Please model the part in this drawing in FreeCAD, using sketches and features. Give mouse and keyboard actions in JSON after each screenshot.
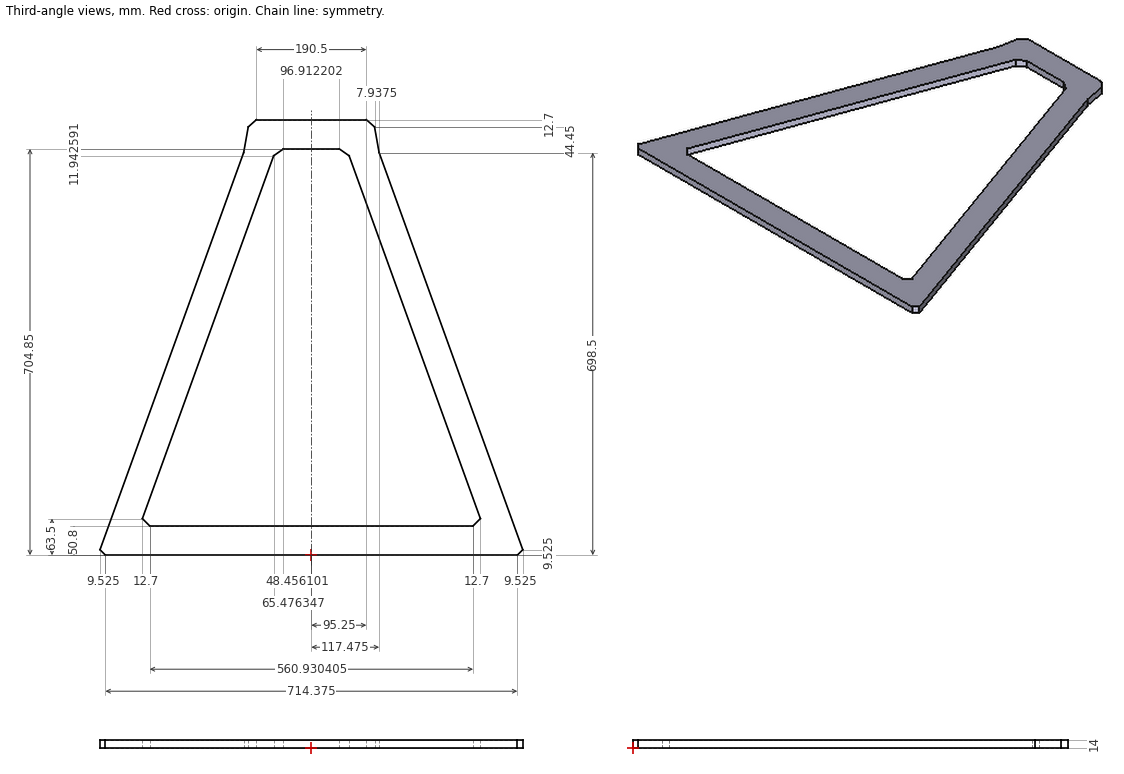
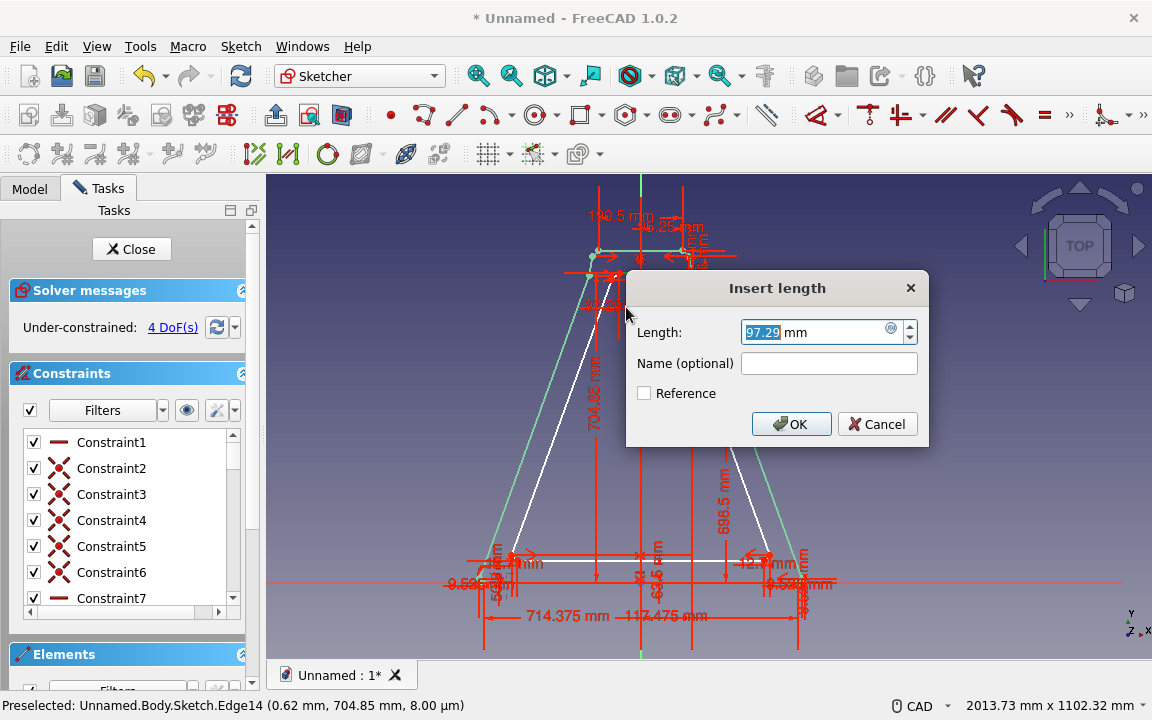
{"action": "type", "text": "96.912202"}
{"action": "key", "text": "Return"}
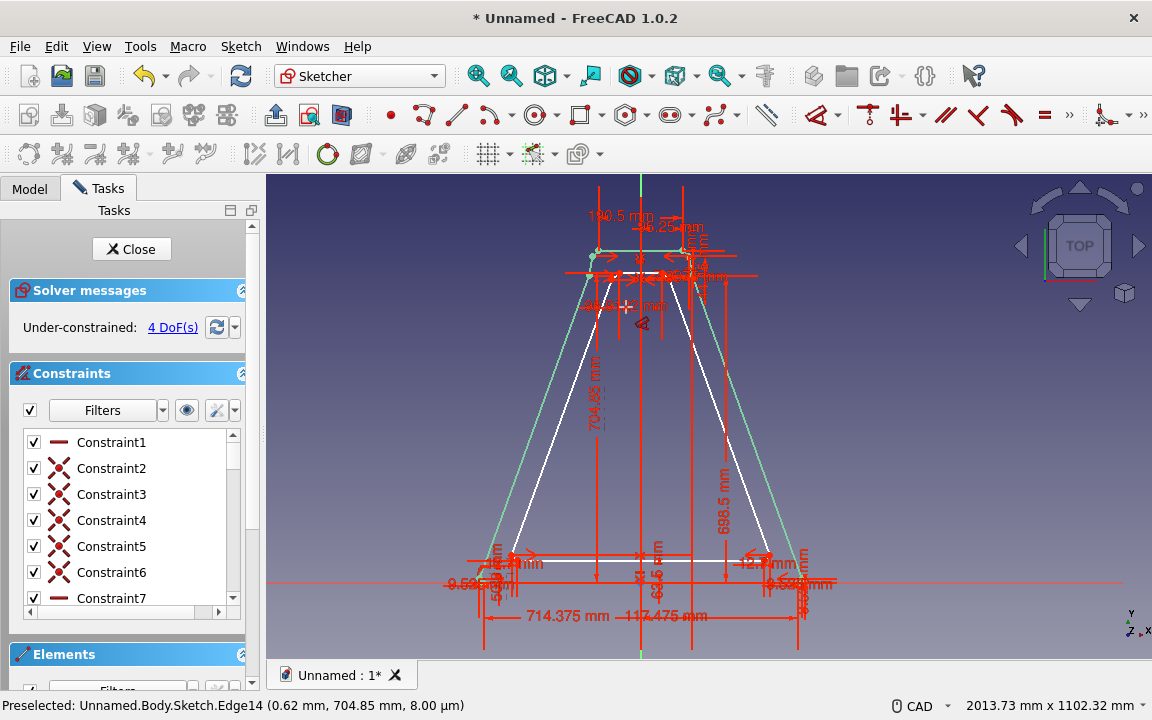
{"action": "left_click", "coordinate": [690, 561]}
{"action": "left_click", "coordinate": [584, 527]}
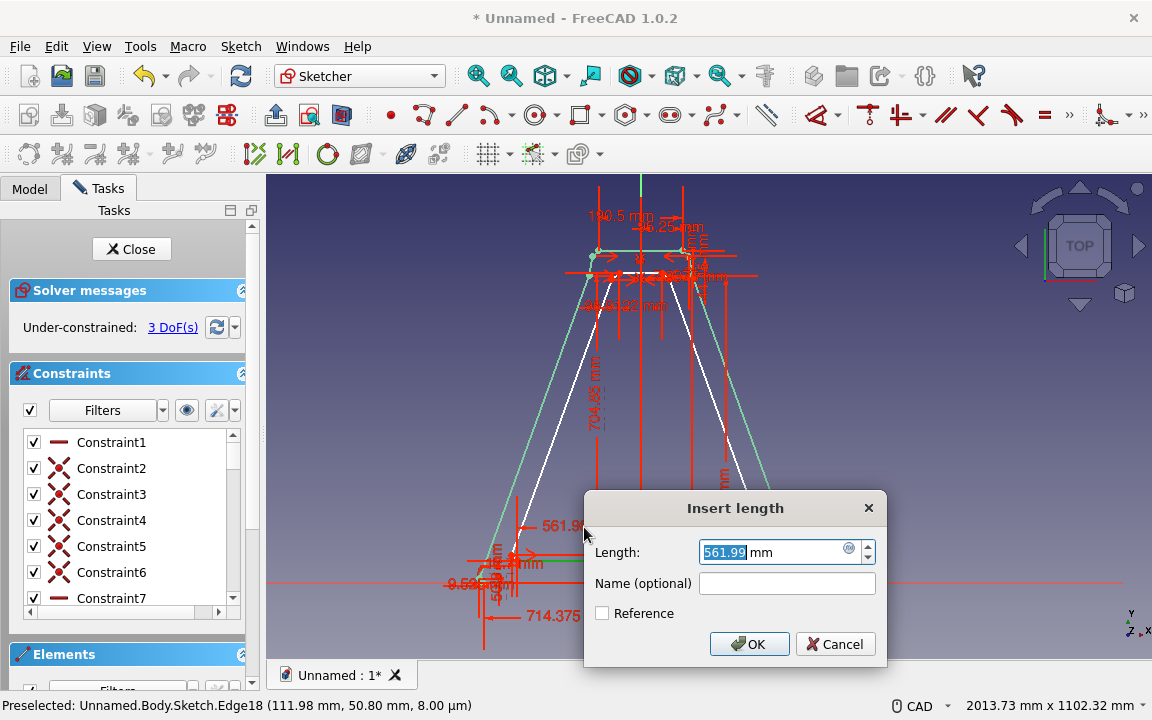
{"action": "type", "text": "560.930405"}
{"action": "key", "text": "Return"}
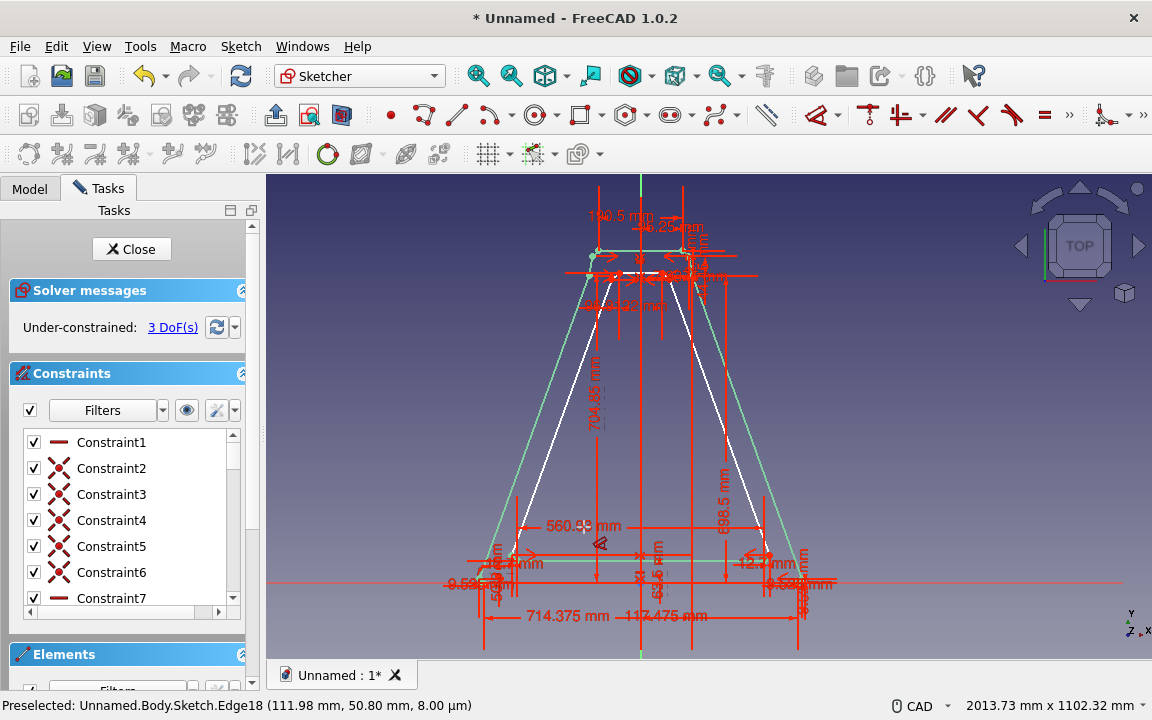
{"action": "scroll", "coordinate": [612, 280], "scroll_direction": "up", "scroll_amount": 2}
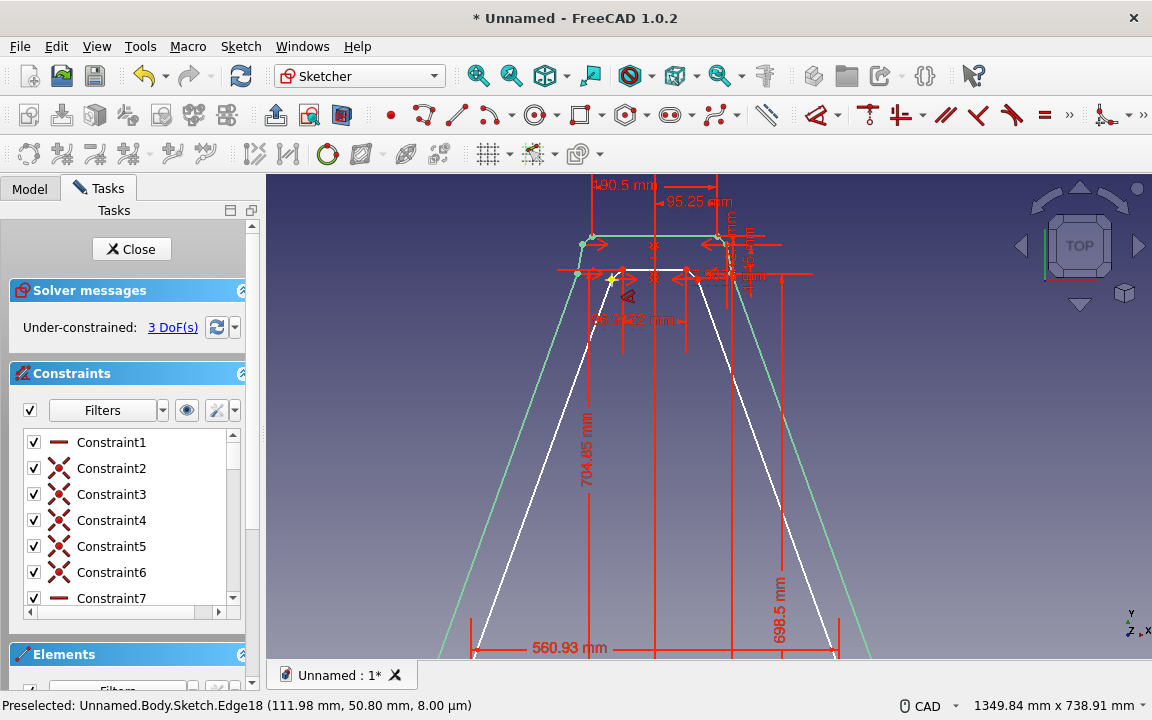
{"action": "left_click", "coordinate": [612, 279]}
{"action": "left_click", "coordinate": [623, 221]}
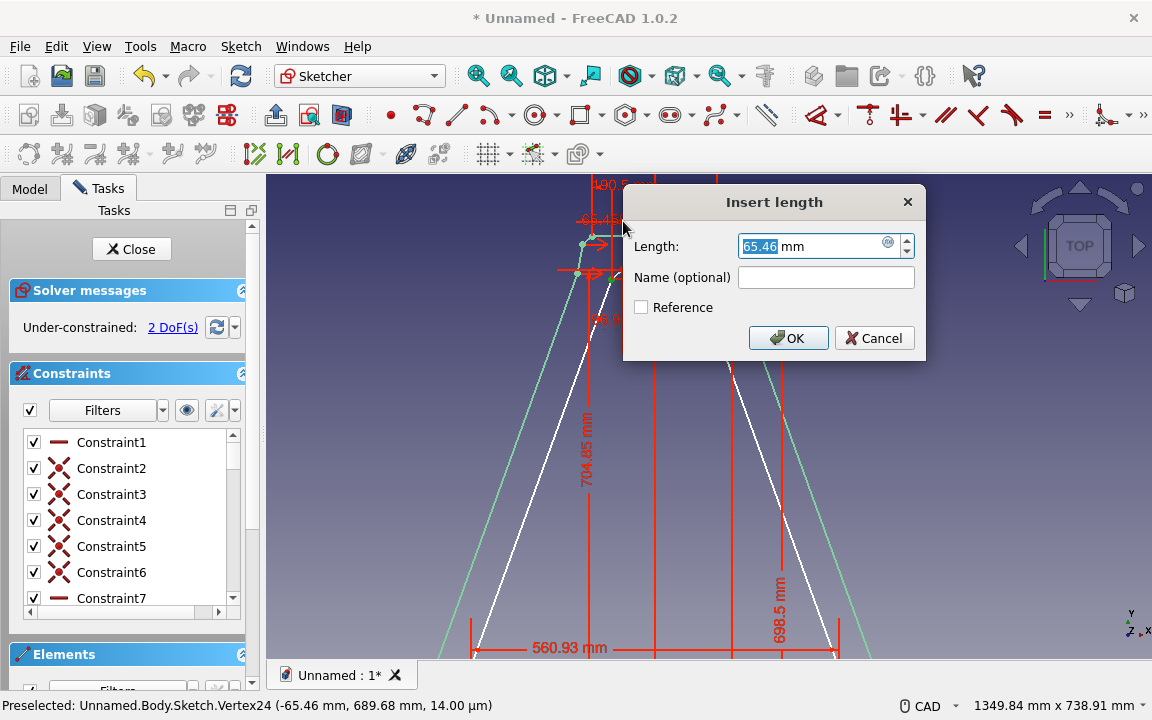
{"action": "type", "text": "65.476347"}
{"action": "key", "text": "Return"}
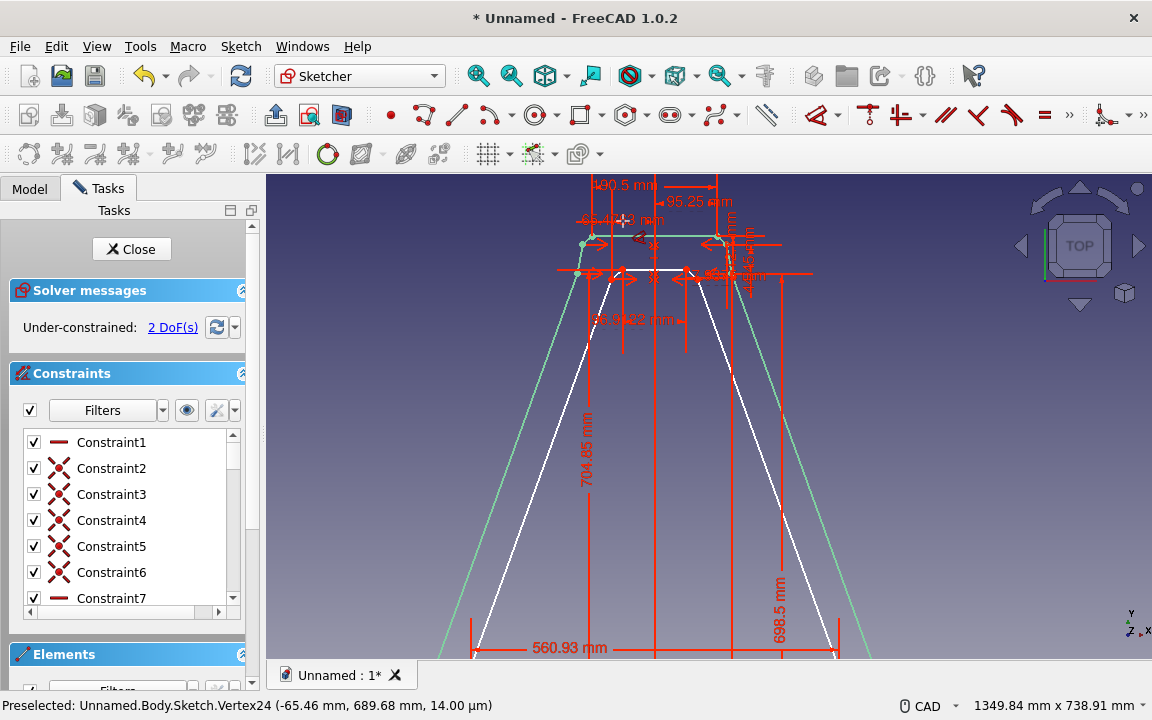
{"action": "scroll", "coordinate": [623, 270], "scroll_direction": "up", "scroll_amount": 2}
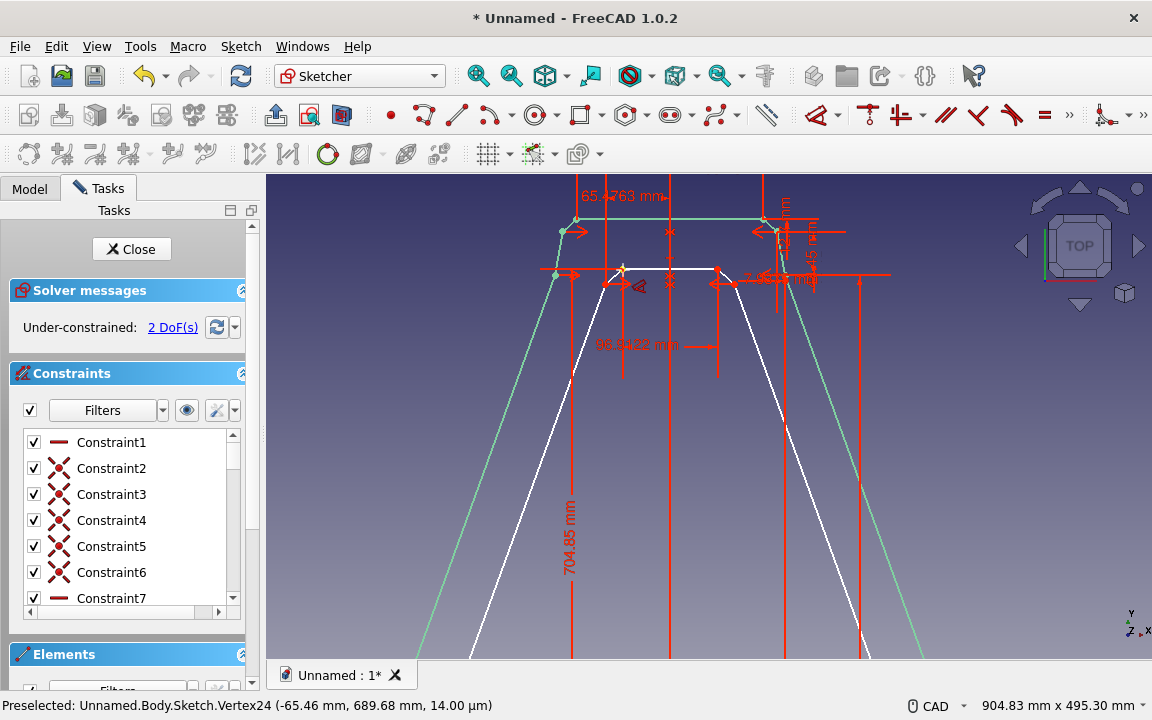
{"action": "left_click", "coordinate": [623, 269]}
{"action": "left_click", "coordinate": [646, 235]}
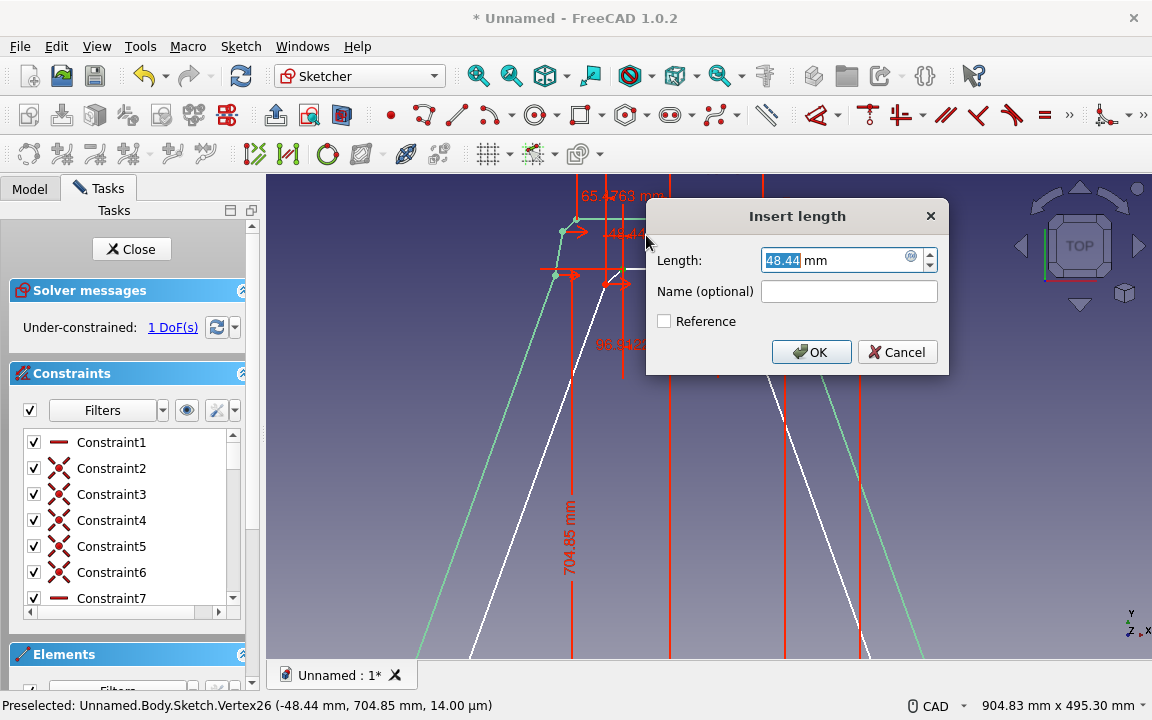
{"action": "type", "text": "48.456101"}
{"action": "key", "text": "Return"}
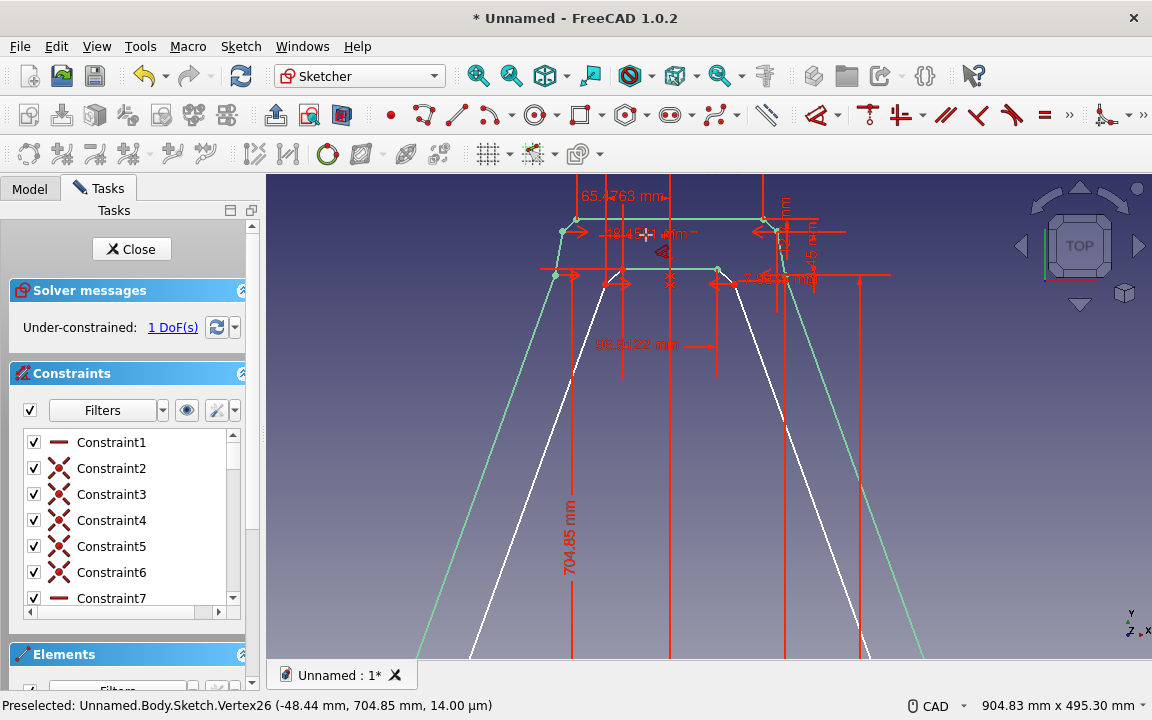
{"action": "scroll", "coordinate": [614, 277], "scroll_direction": "up", "scroll_amount": 7}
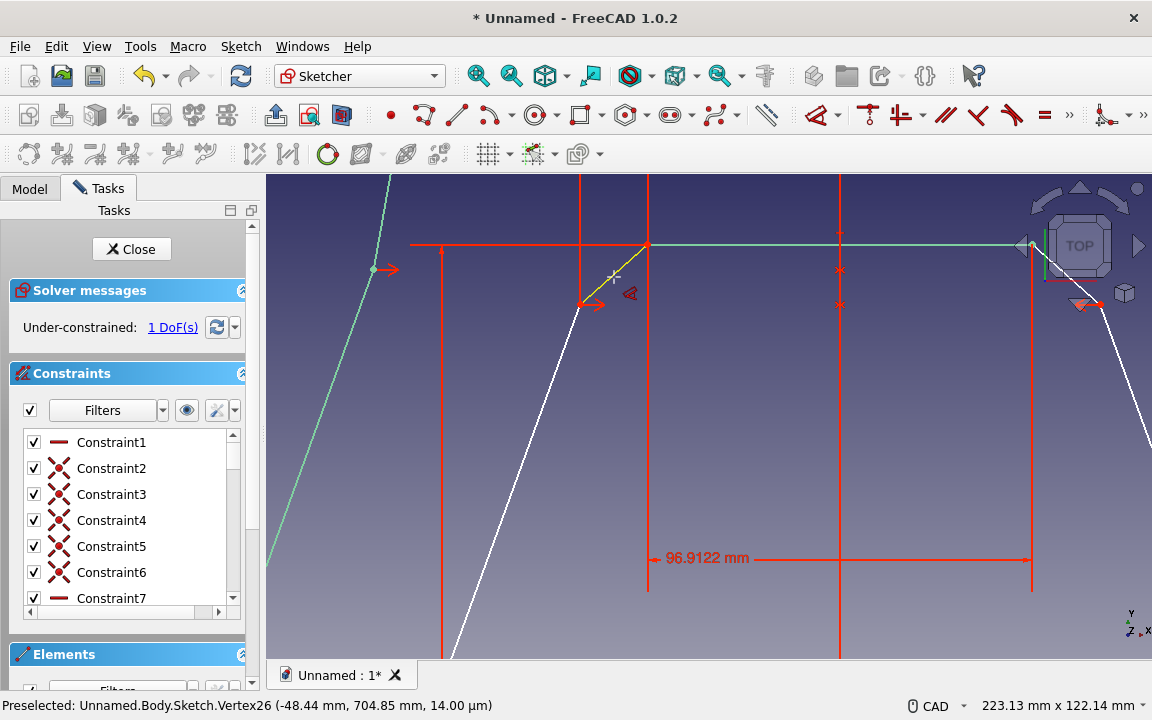
{"action": "left_click", "coordinate": [614, 275]}
{"action": "left_click", "coordinate": [546, 275]}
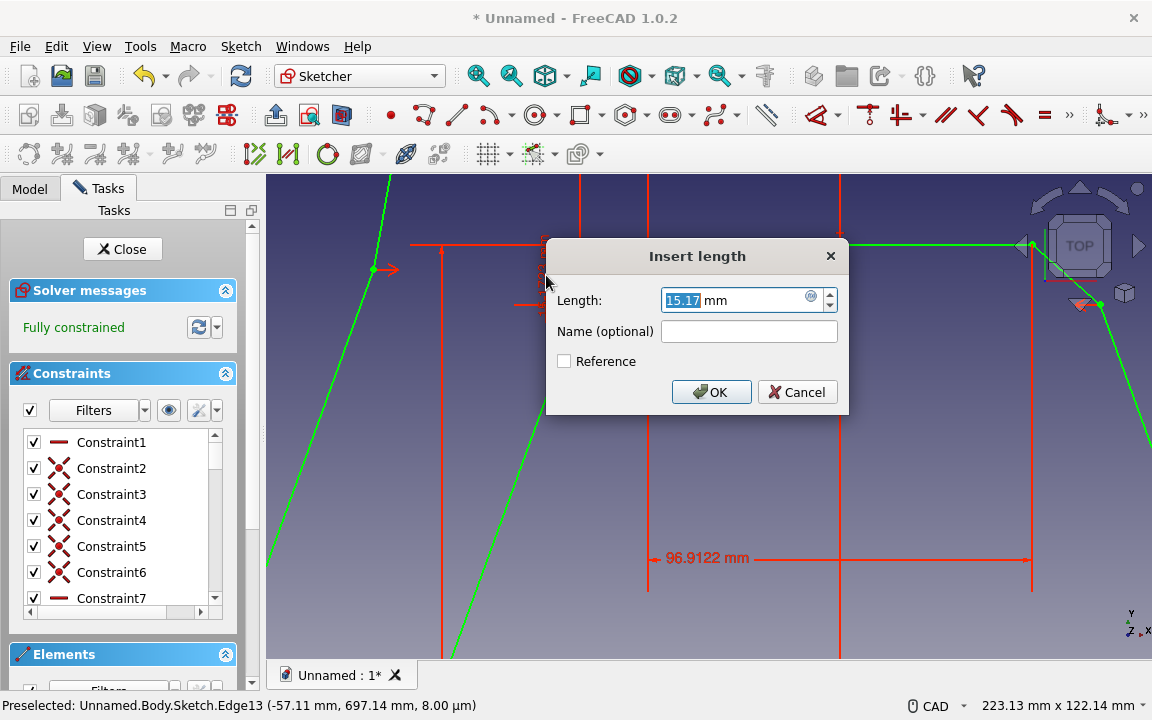
{"action": "type", "text": "11.942591"}
{"action": "key", "text": "Return"}
{"action": "key", "text": "Escape"}